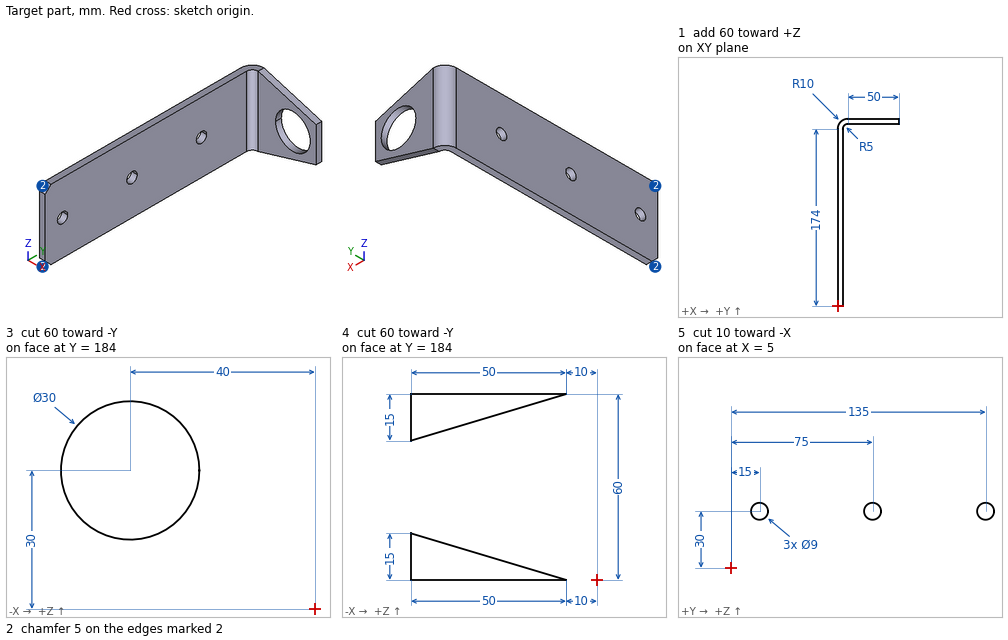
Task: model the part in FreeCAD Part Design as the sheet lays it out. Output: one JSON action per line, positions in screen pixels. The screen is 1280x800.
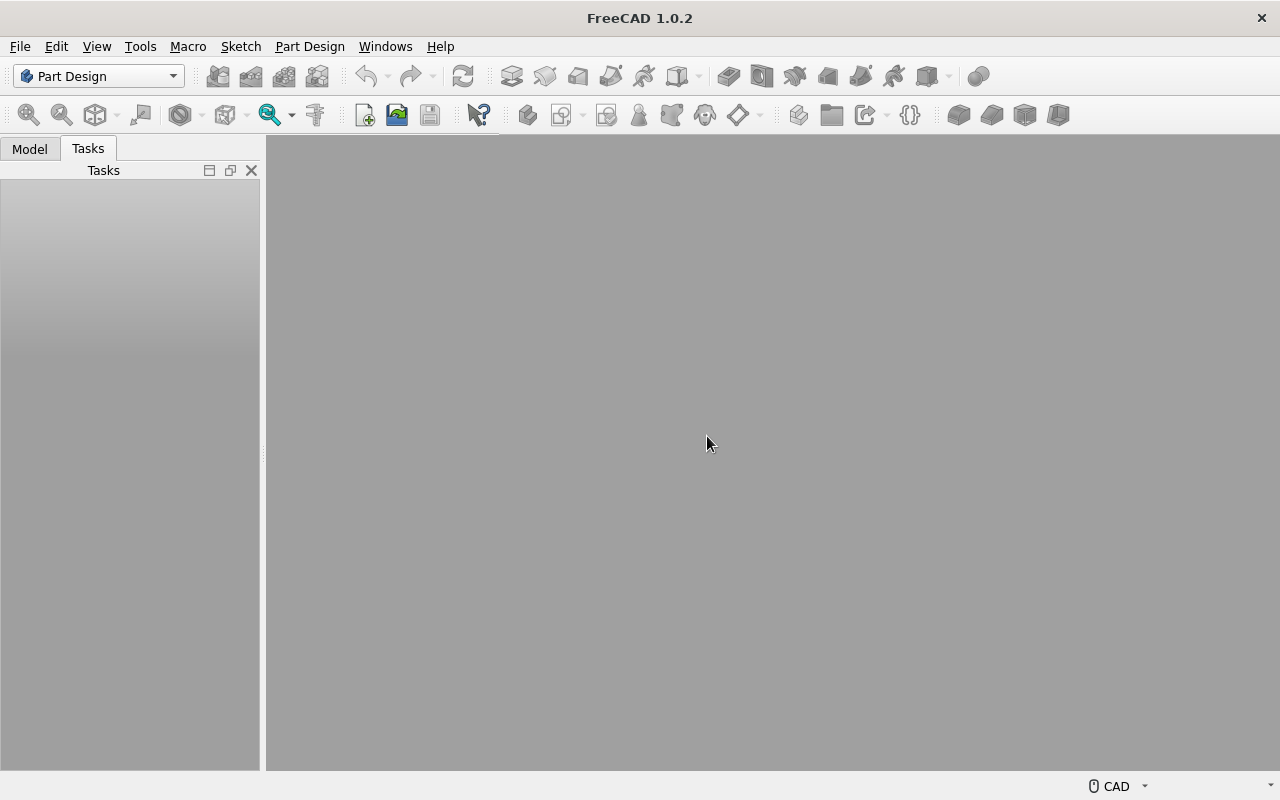
{"action": "left_click", "coordinate": [364, 116]}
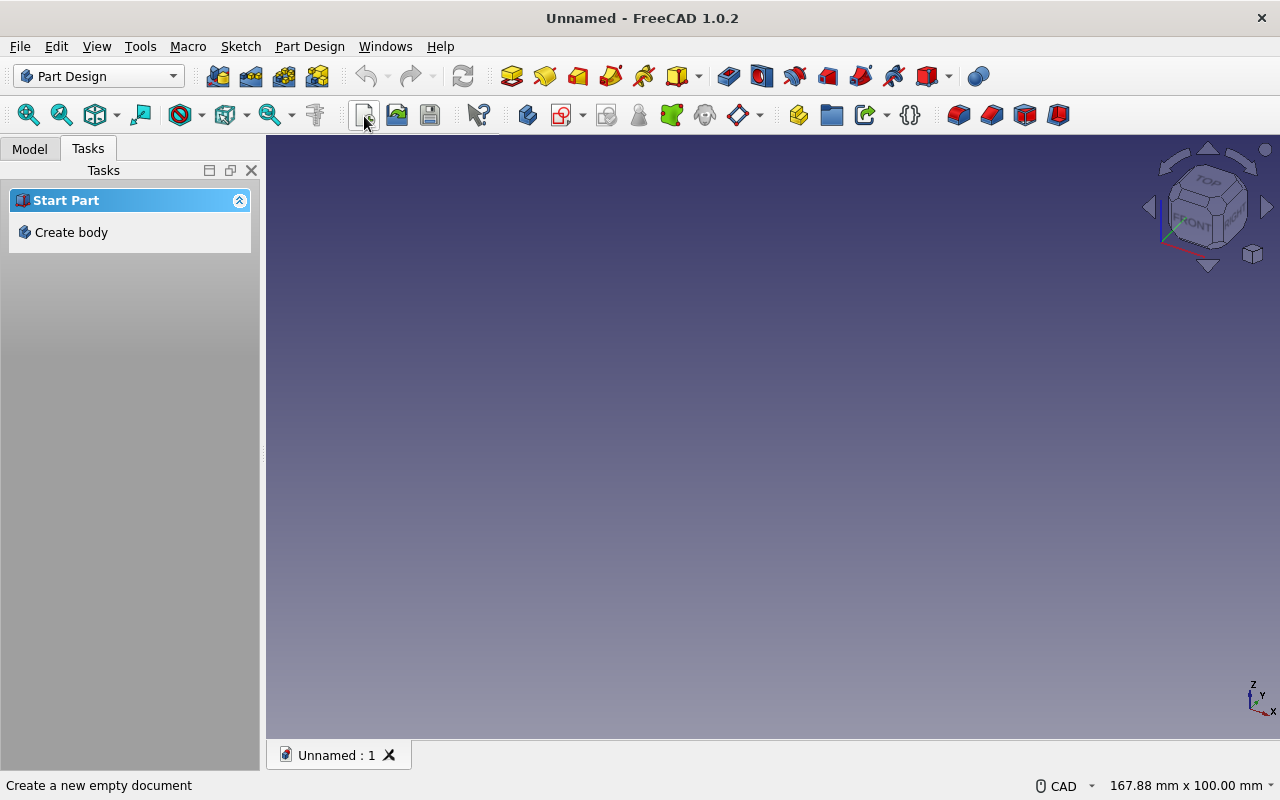
{"action": "left_click", "coordinate": [560, 116]}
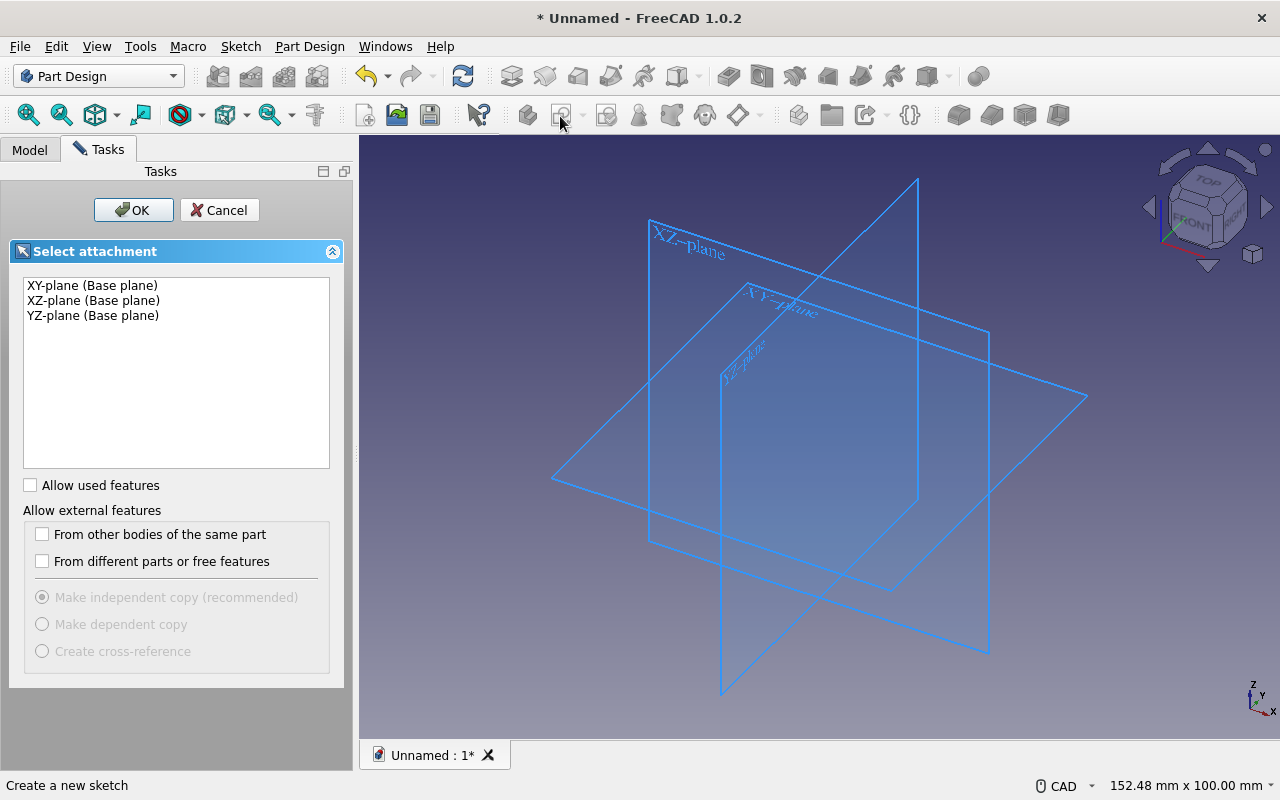
{"action": "left_click", "coordinate": [84, 286]}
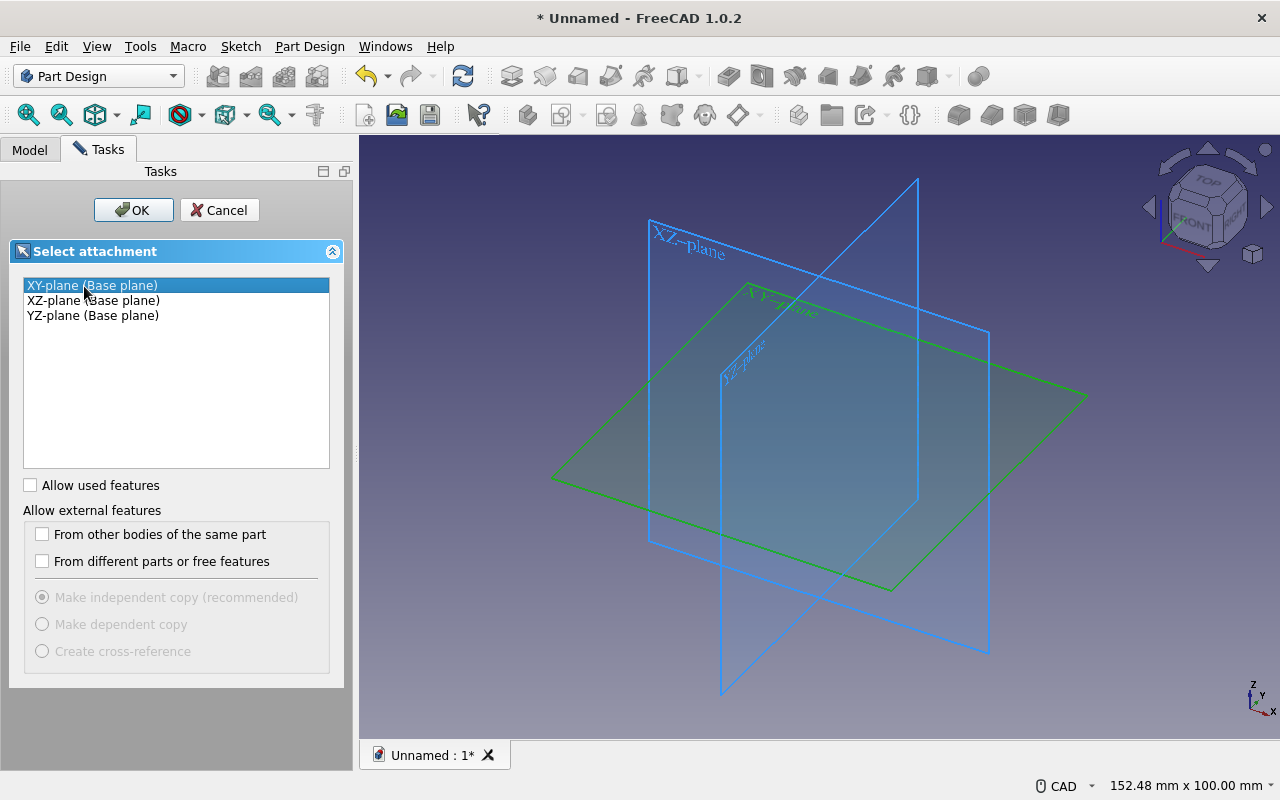
{"action": "left_click", "coordinate": [134, 210]}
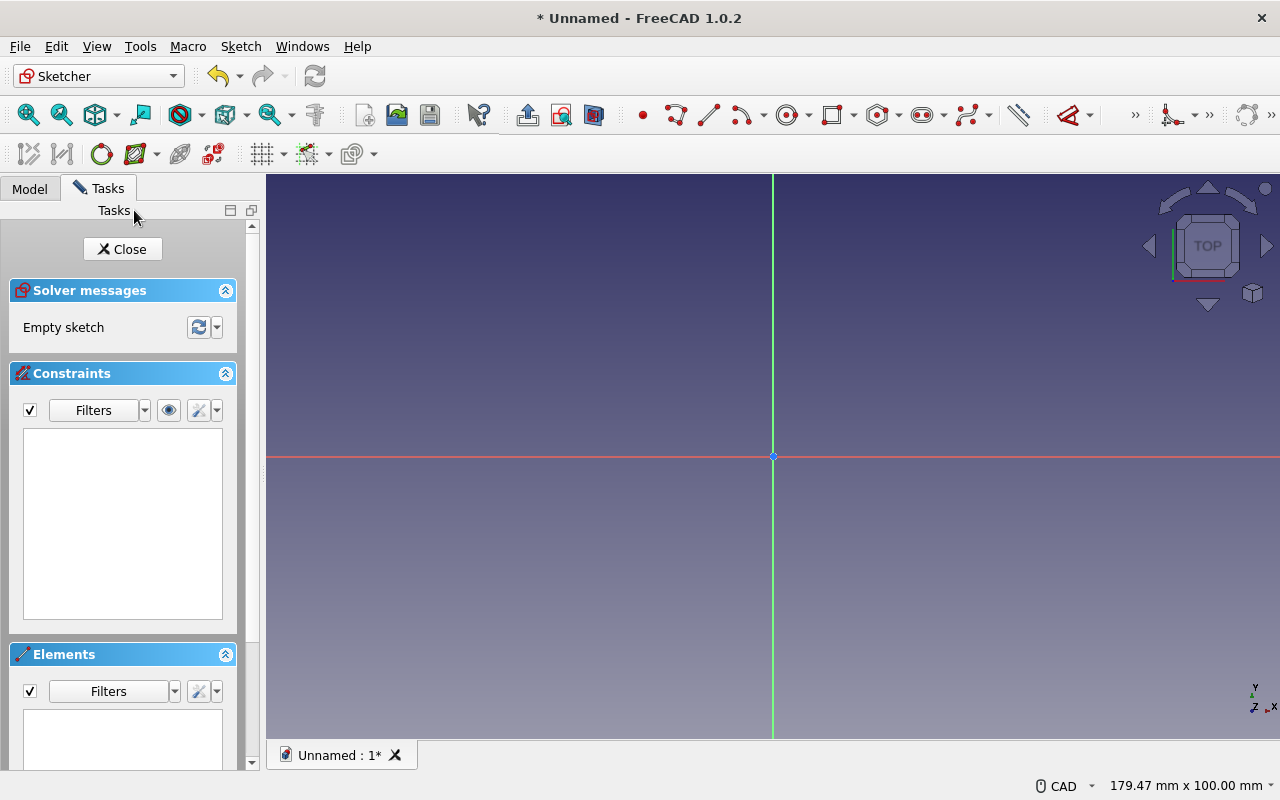
{"action": "scroll", "coordinate": [566, 711], "scroll_direction": "down", "scroll_amount": 5}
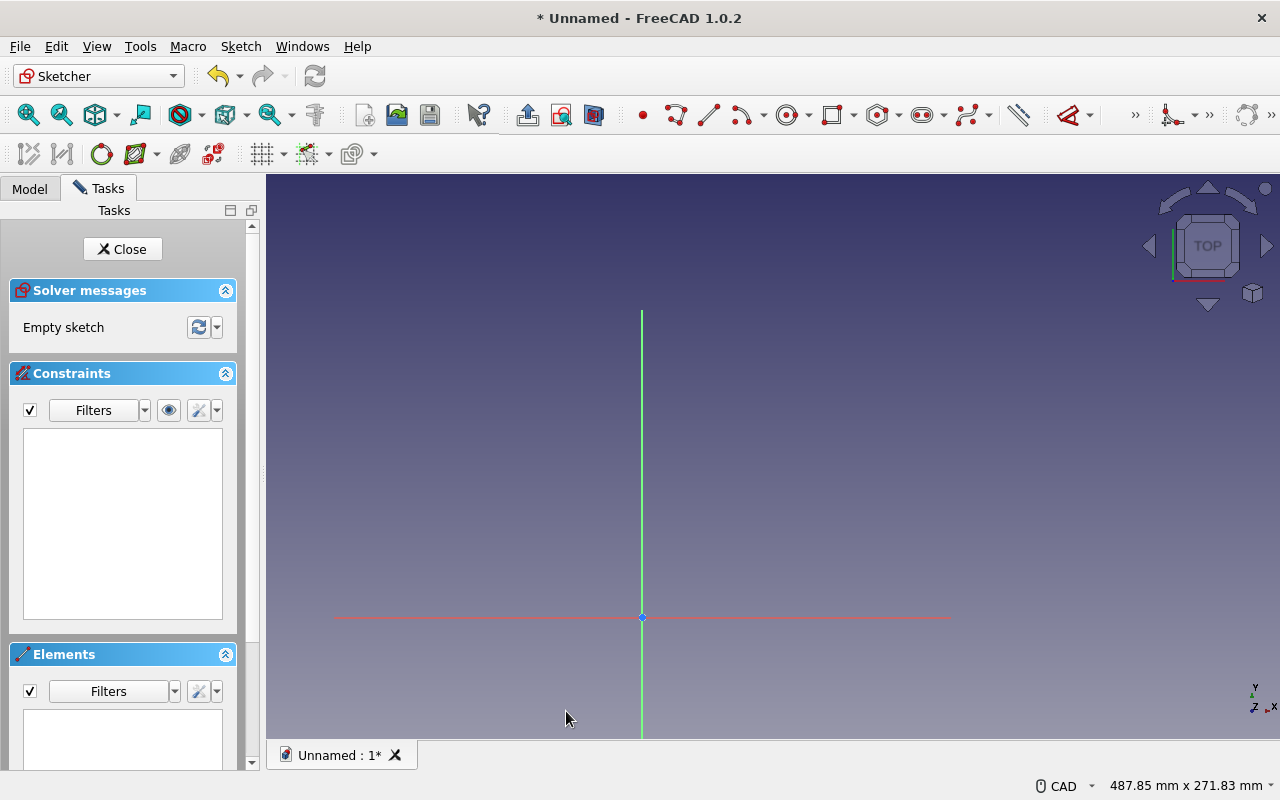
{"action": "left_click", "coordinate": [676, 116]}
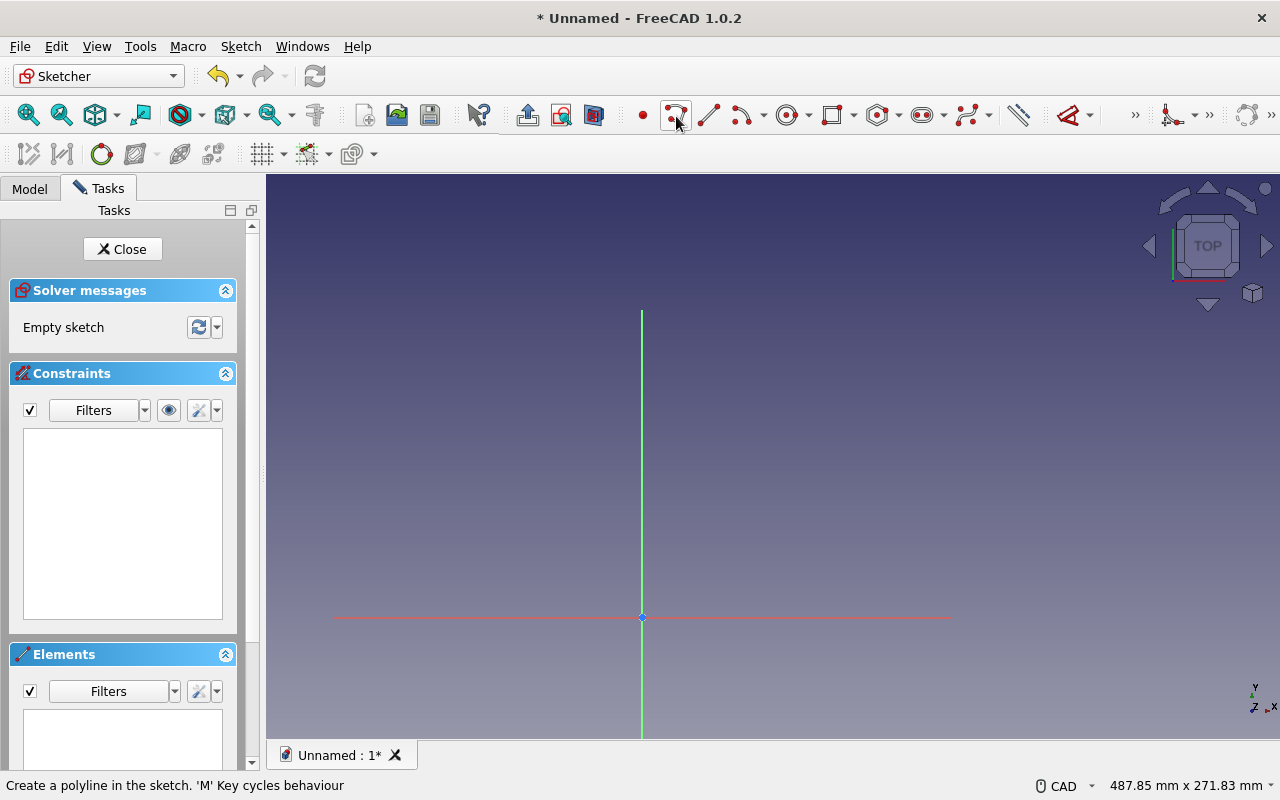
{"action": "left_click", "coordinate": [642, 256]}
{"action": "left_click", "coordinate": [642, 618]}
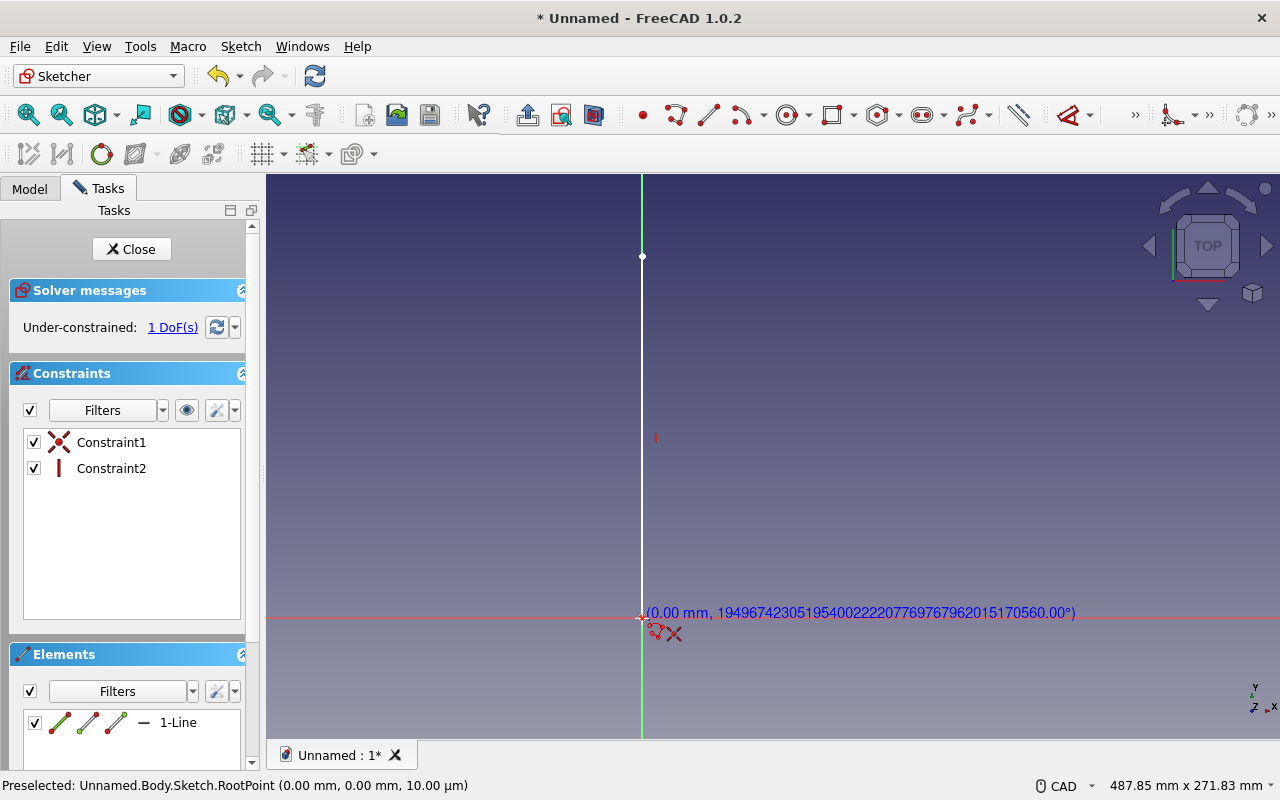
{"action": "scroll", "coordinate": [653, 618], "scroll_direction": "up", "scroll_amount": 3}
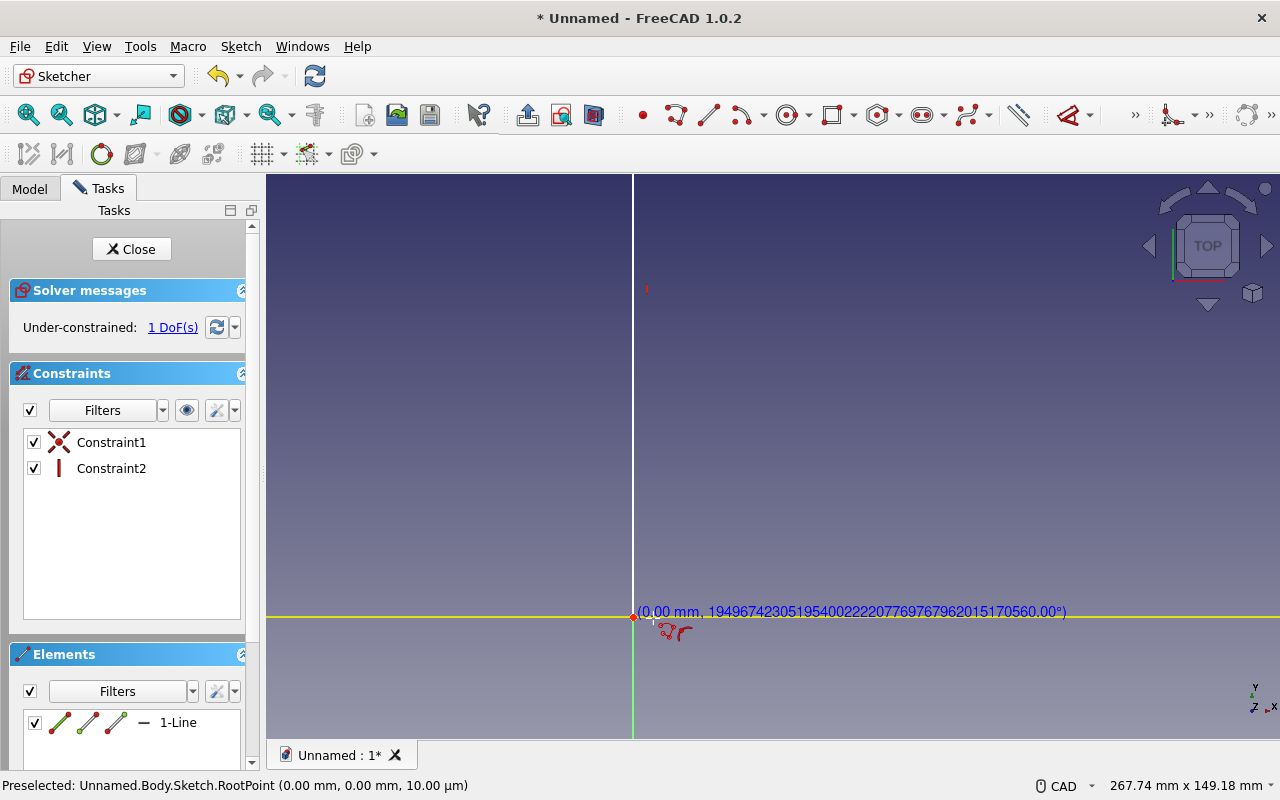
{"action": "left_click", "coordinate": [652, 608]}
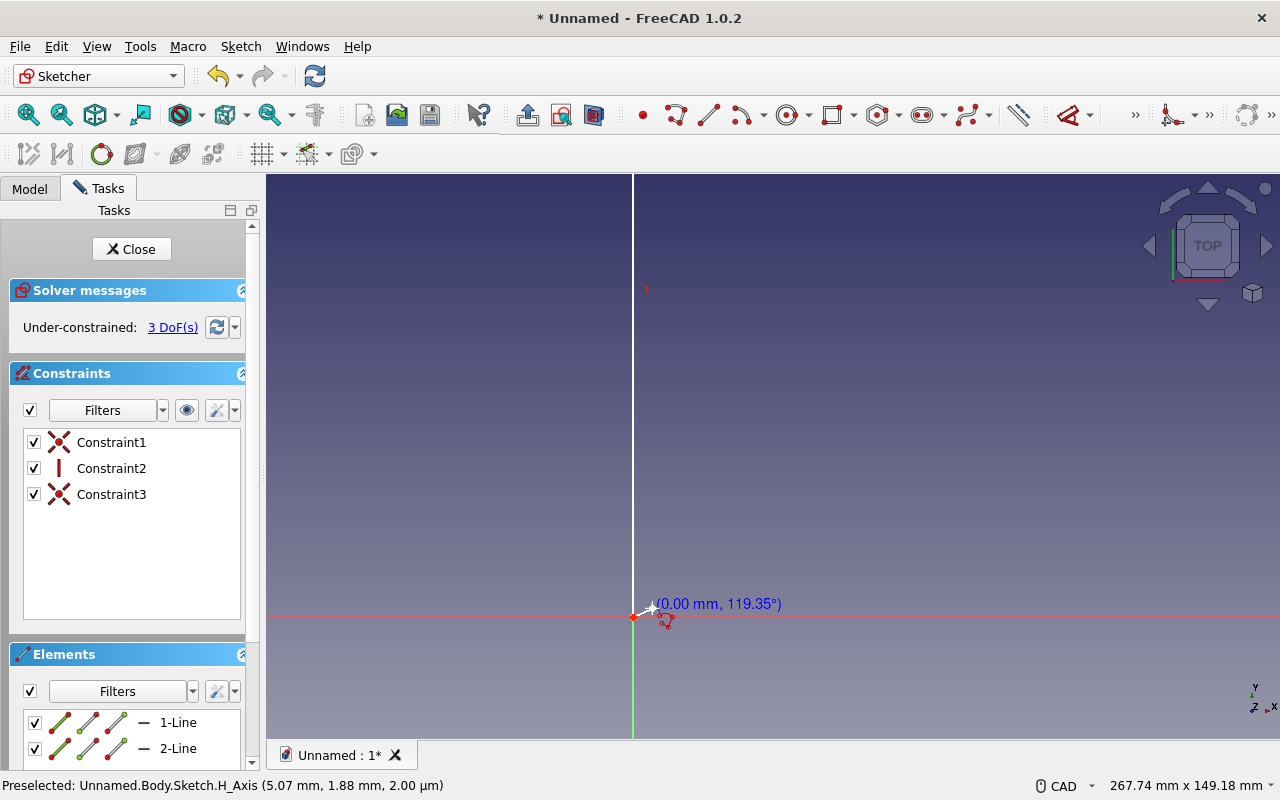
{"action": "scroll", "coordinate": [653, 685], "scroll_direction": "down", "scroll_amount": 3}